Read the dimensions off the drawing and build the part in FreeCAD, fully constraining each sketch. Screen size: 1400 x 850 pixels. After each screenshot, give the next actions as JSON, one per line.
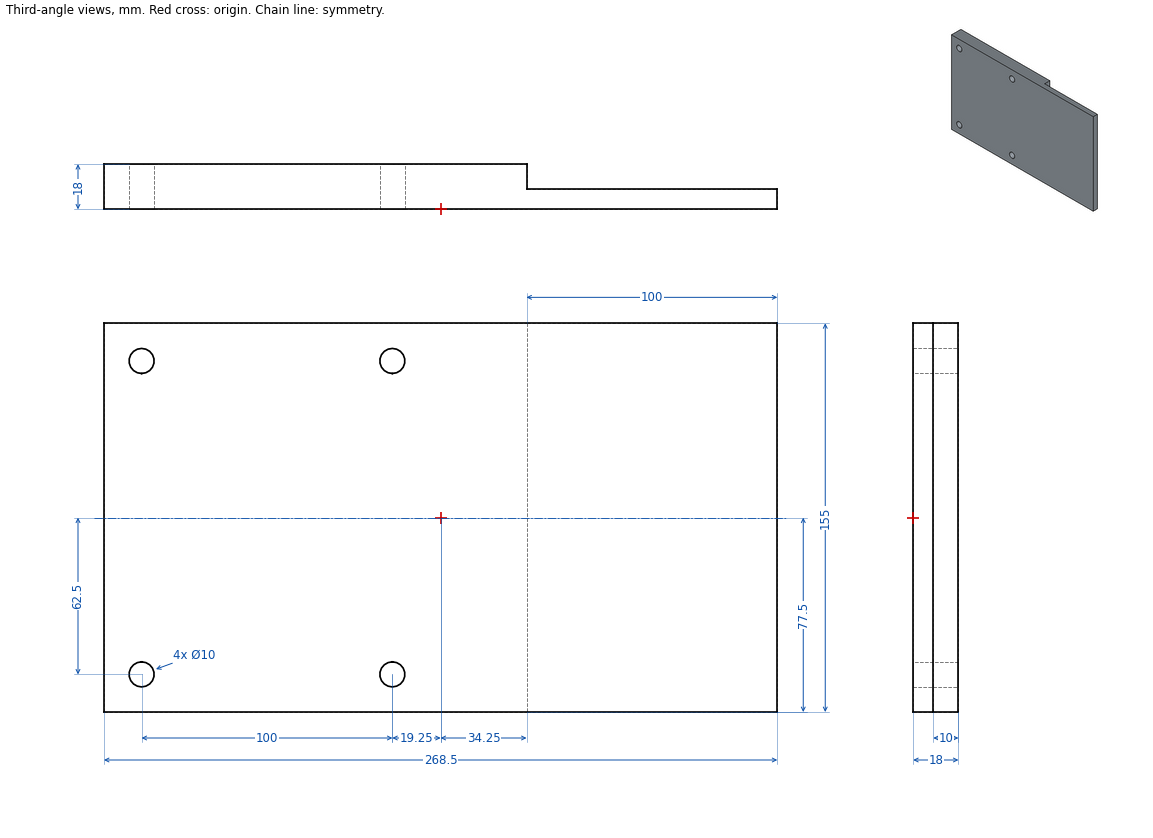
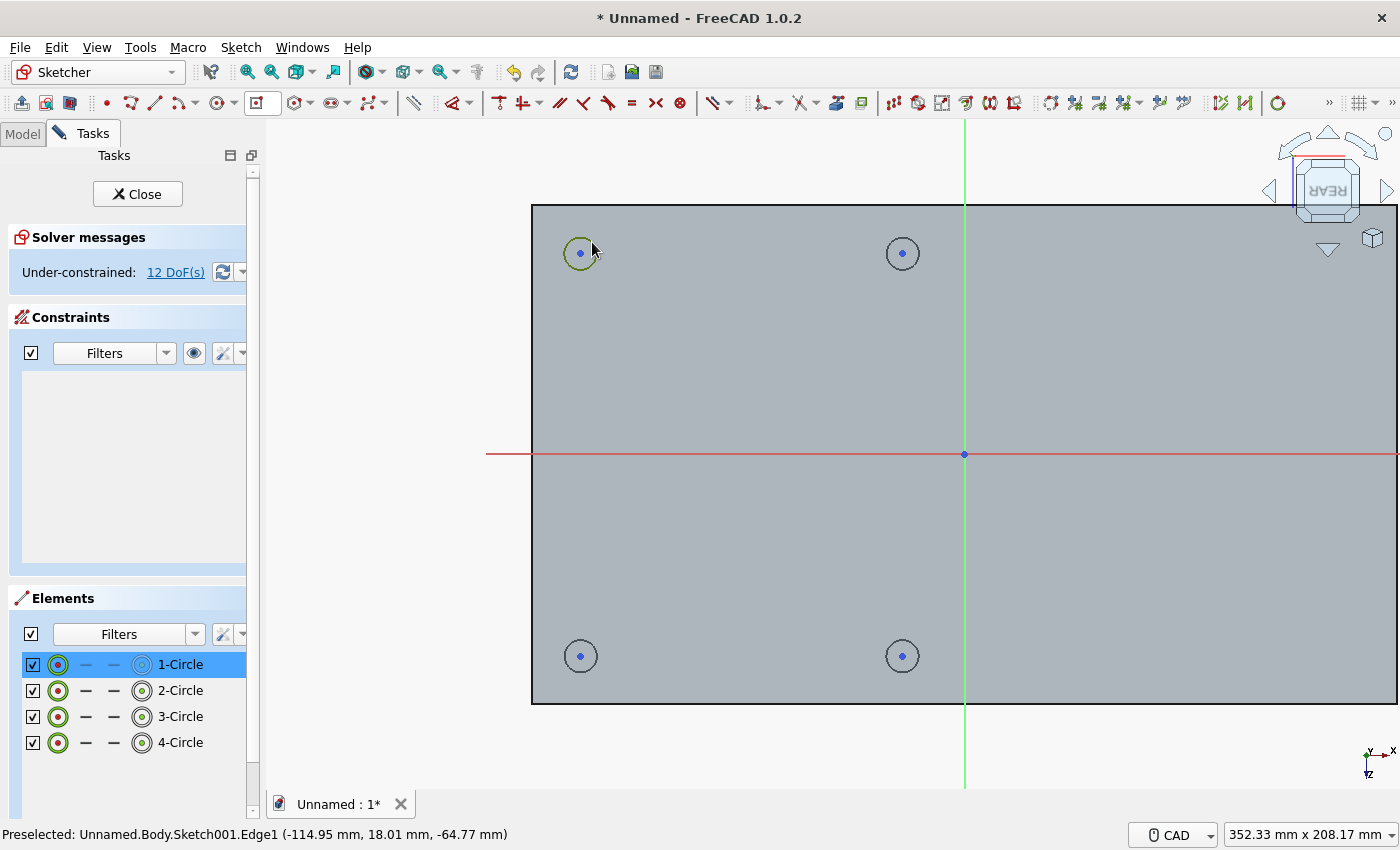
{"action": "left_click", "coordinate": [914, 242]}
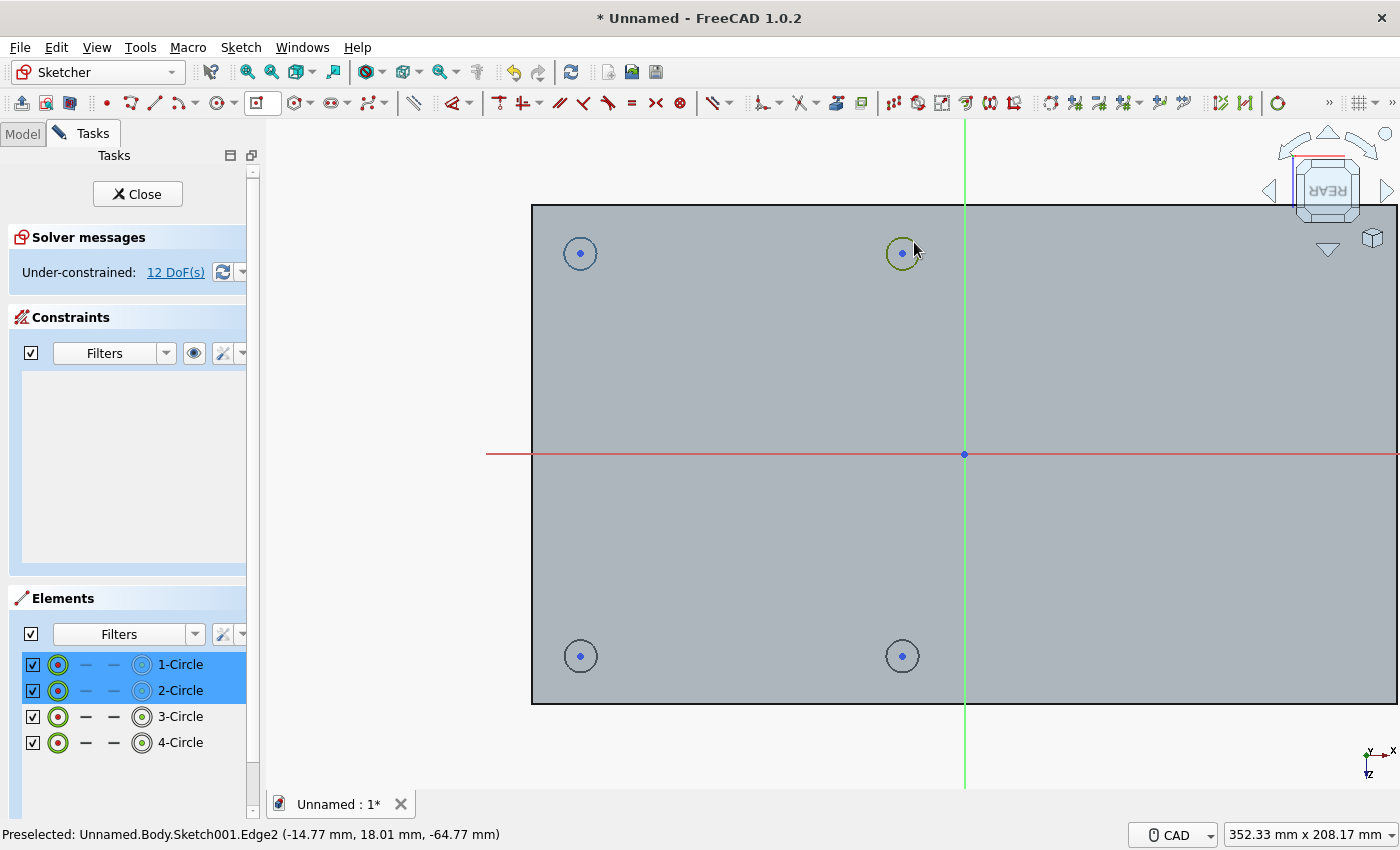
{"action": "left_click", "coordinate": [914, 645]}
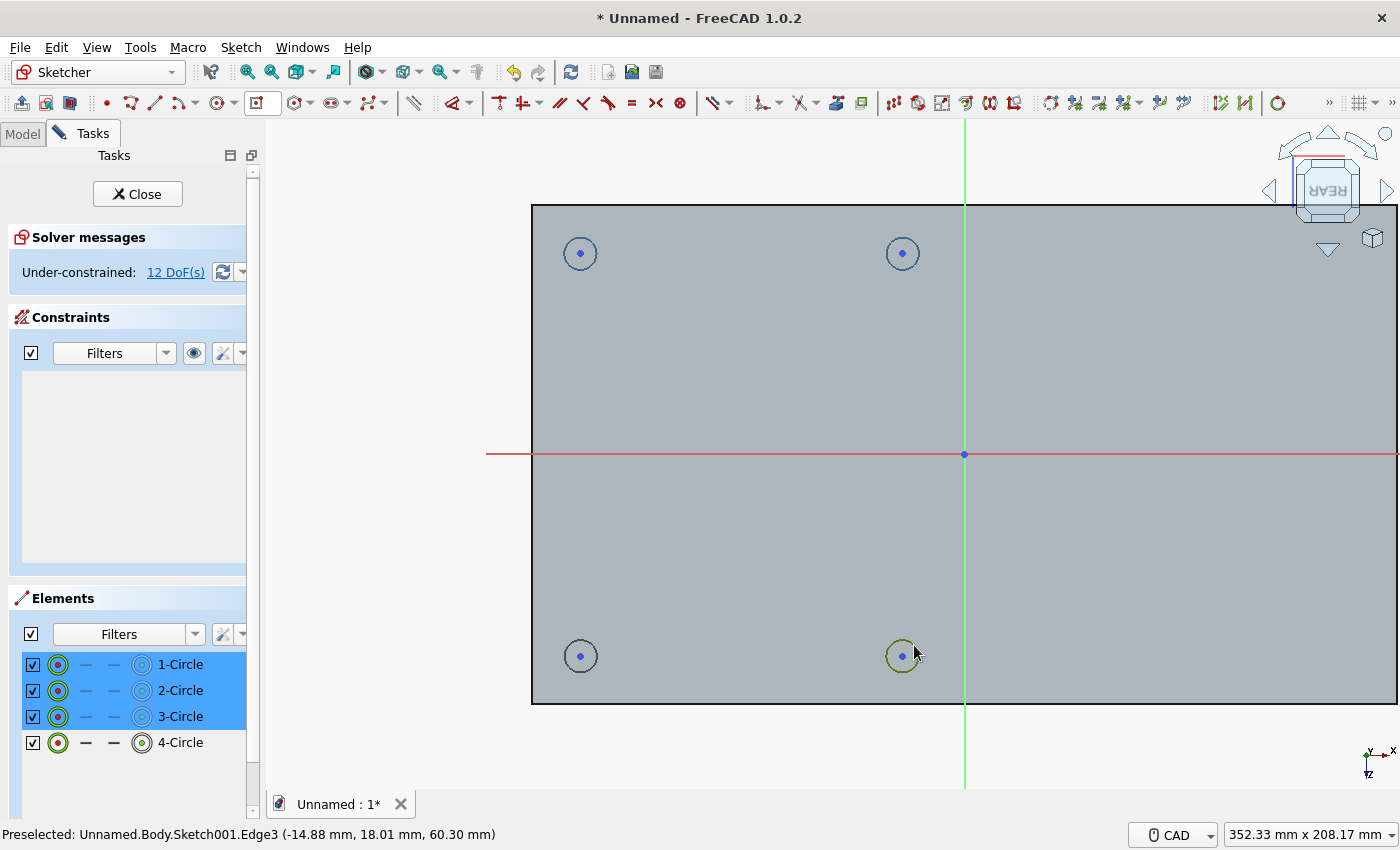
{"action": "left_click", "coordinate": [592, 645]}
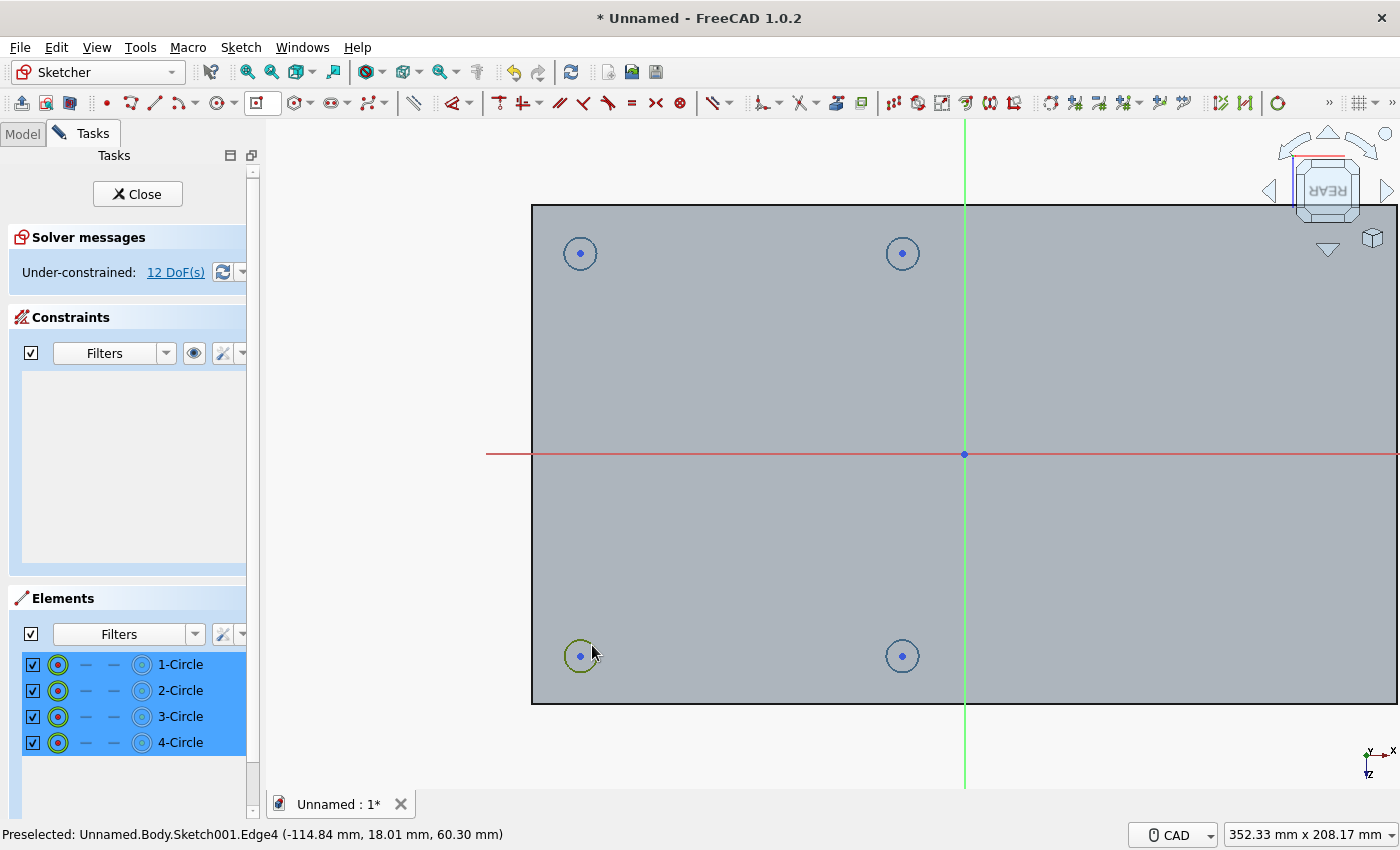
{"action": "key", "text": "e"}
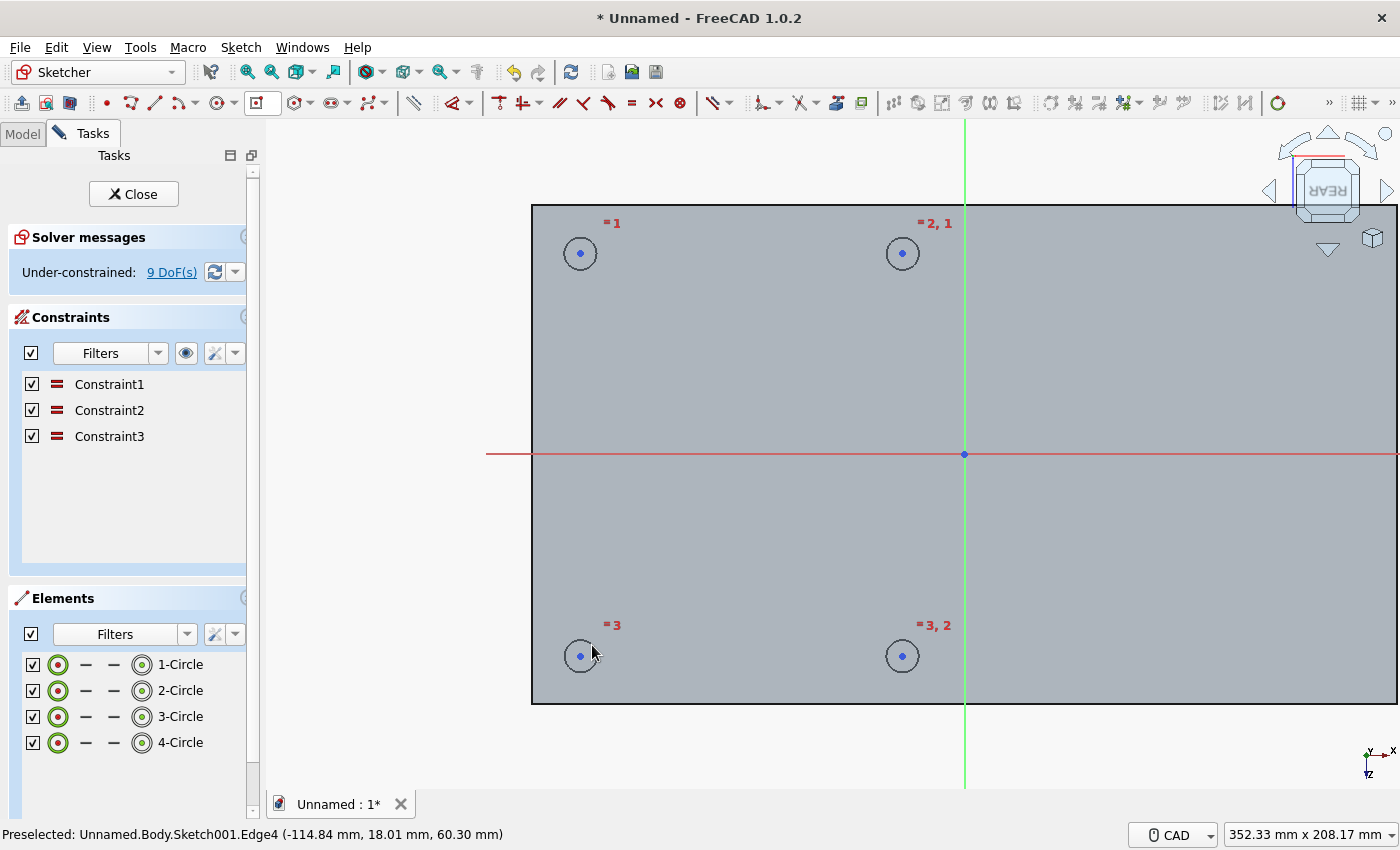
{"action": "left_click", "coordinate": [903, 254]}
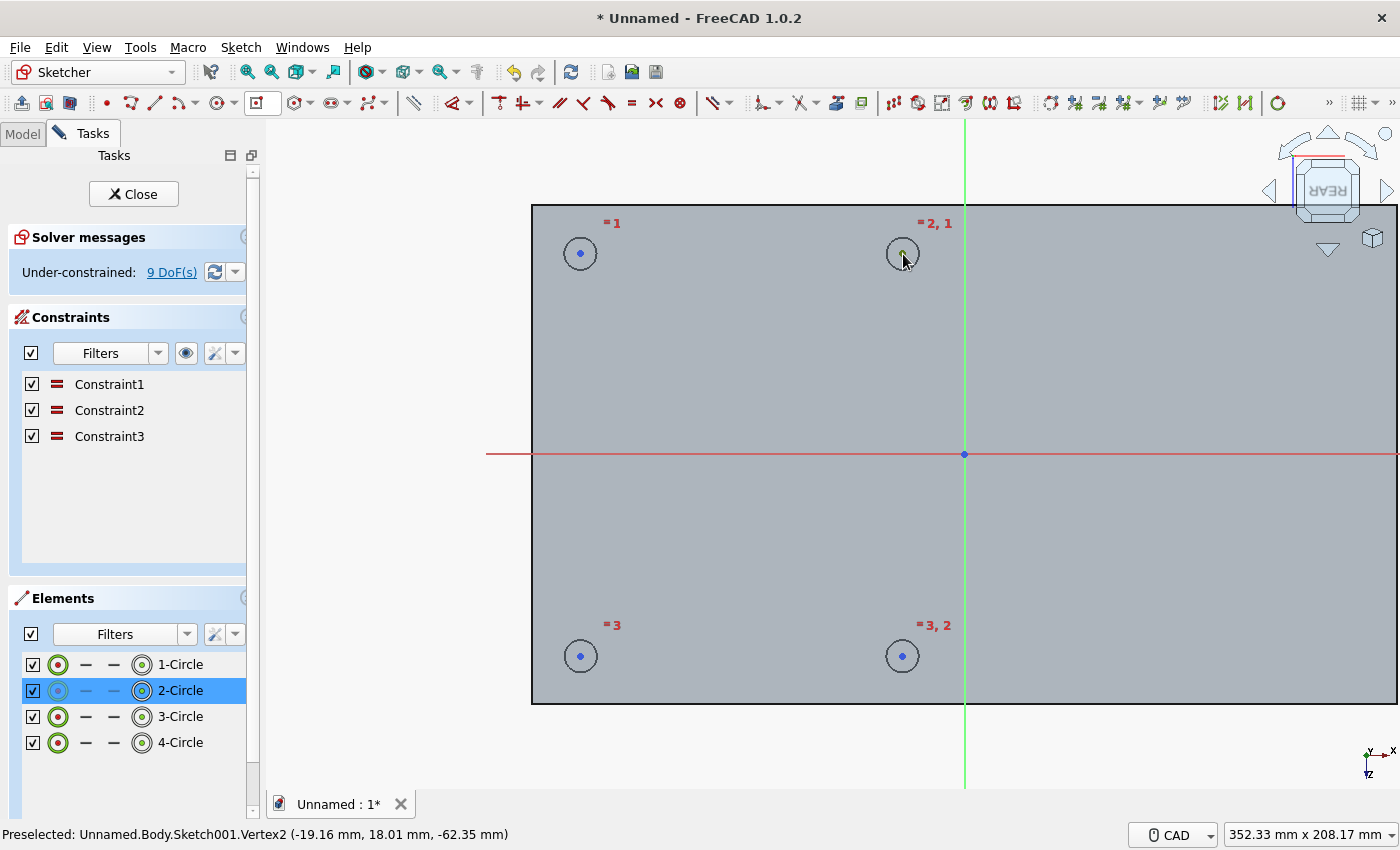
{"action": "left_click", "coordinate": [903, 656]}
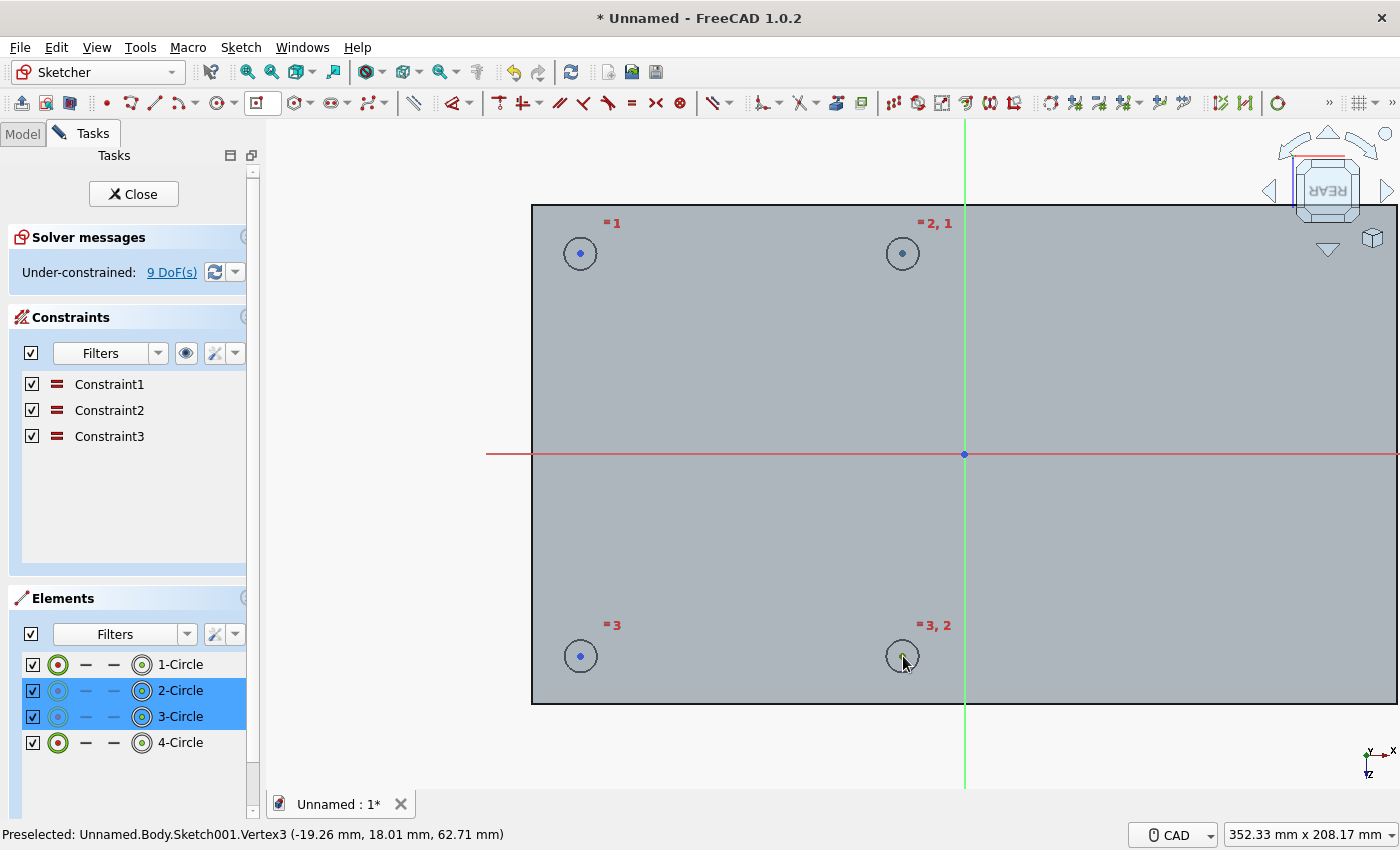
{"action": "left_click", "coordinate": [496, 454]}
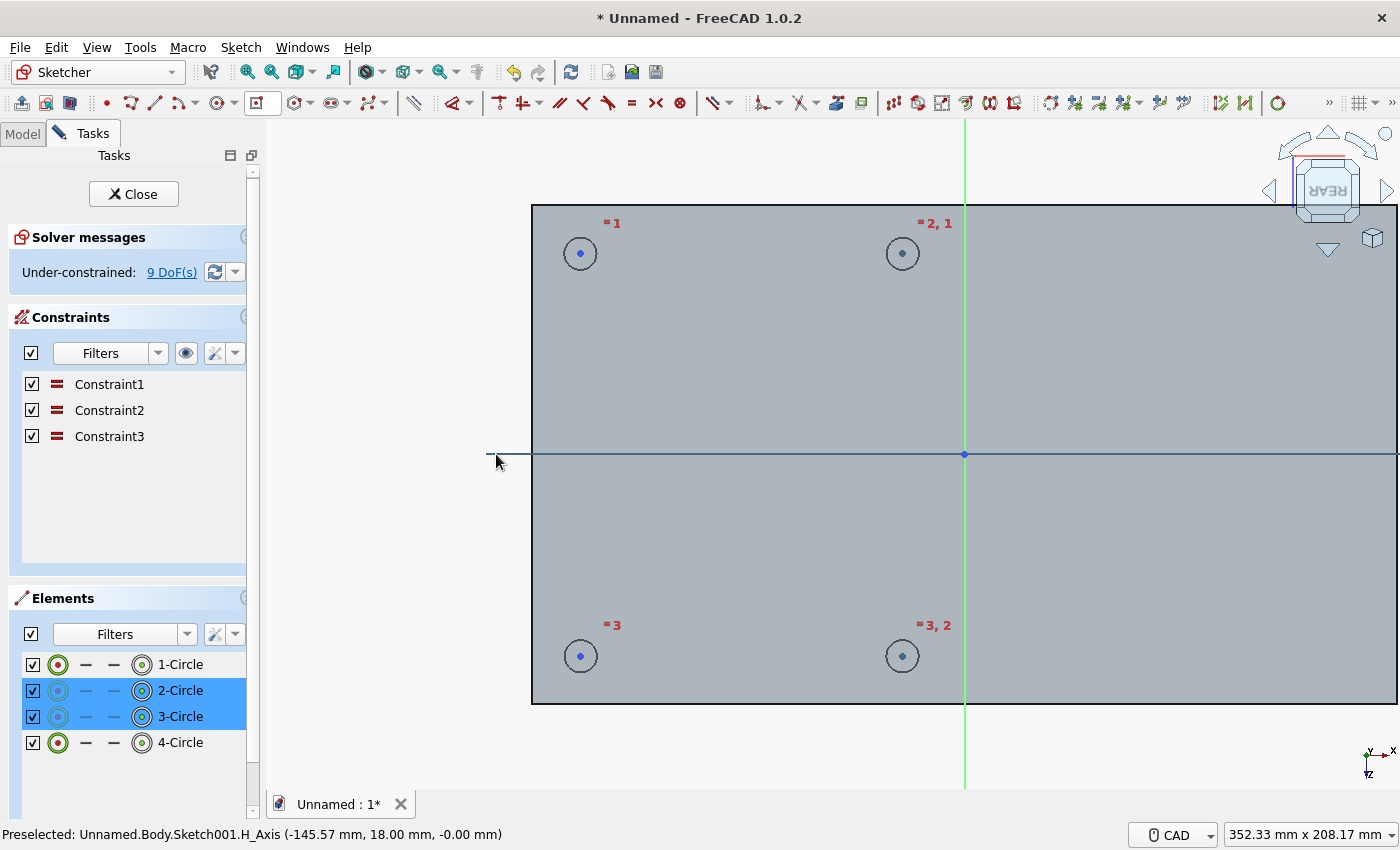
{"action": "key", "text": "s"}